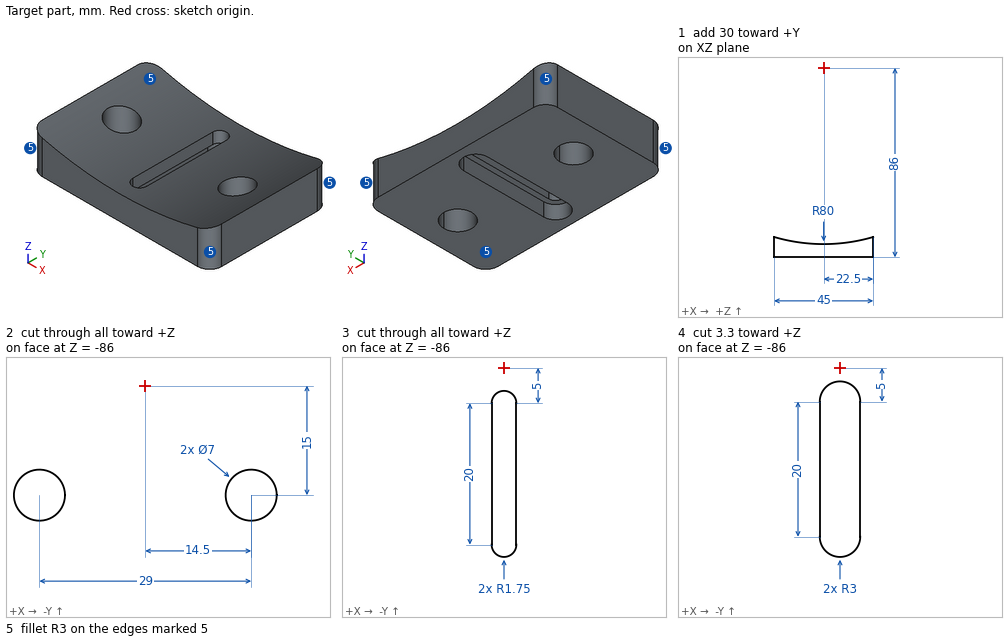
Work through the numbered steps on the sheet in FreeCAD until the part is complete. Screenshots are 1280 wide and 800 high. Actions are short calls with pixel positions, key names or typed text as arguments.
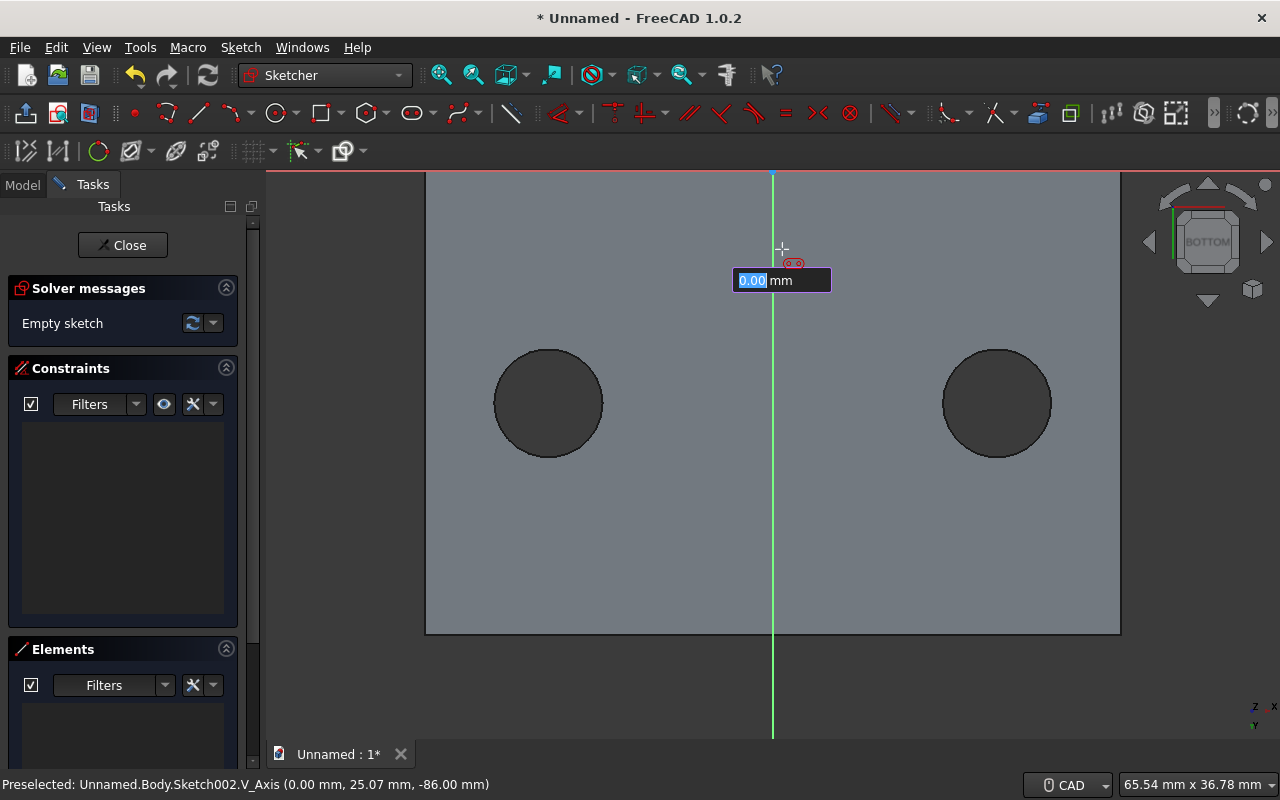
click(746, 403)
key(Escape)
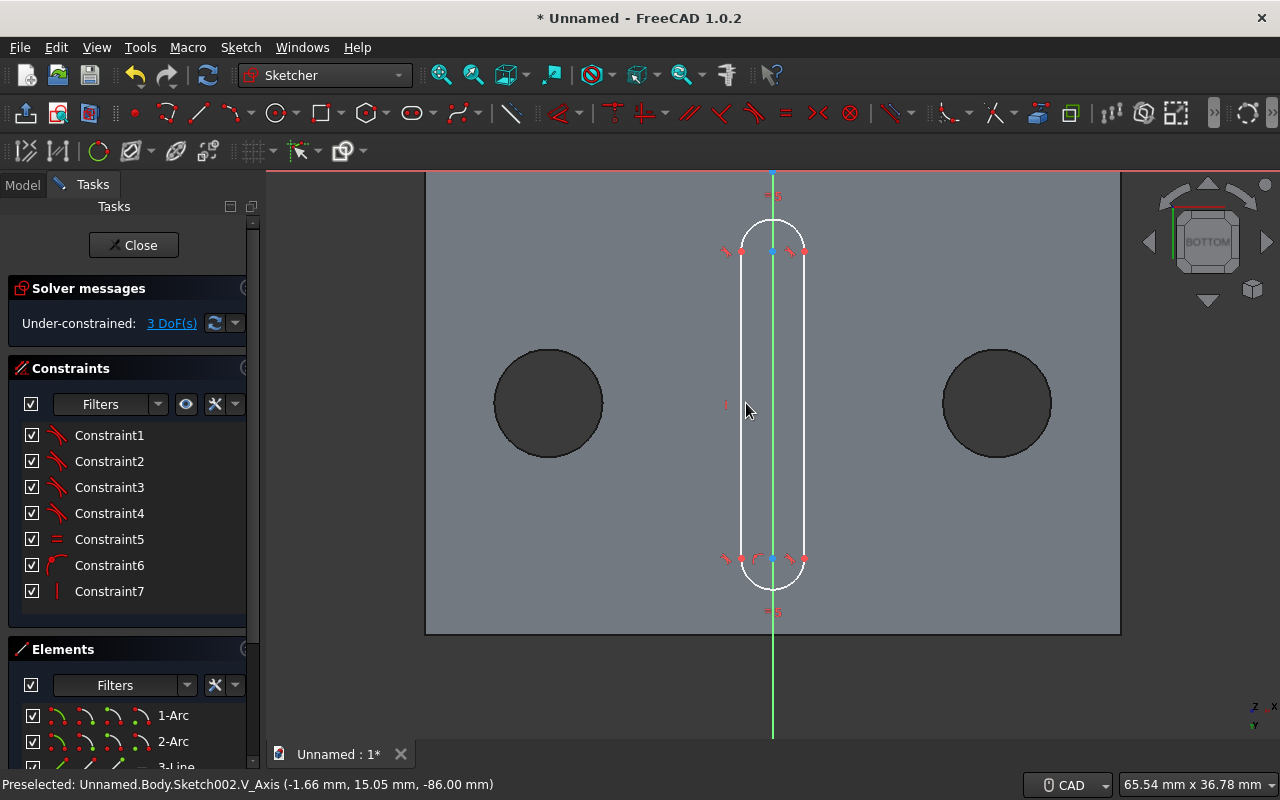
click(558, 114)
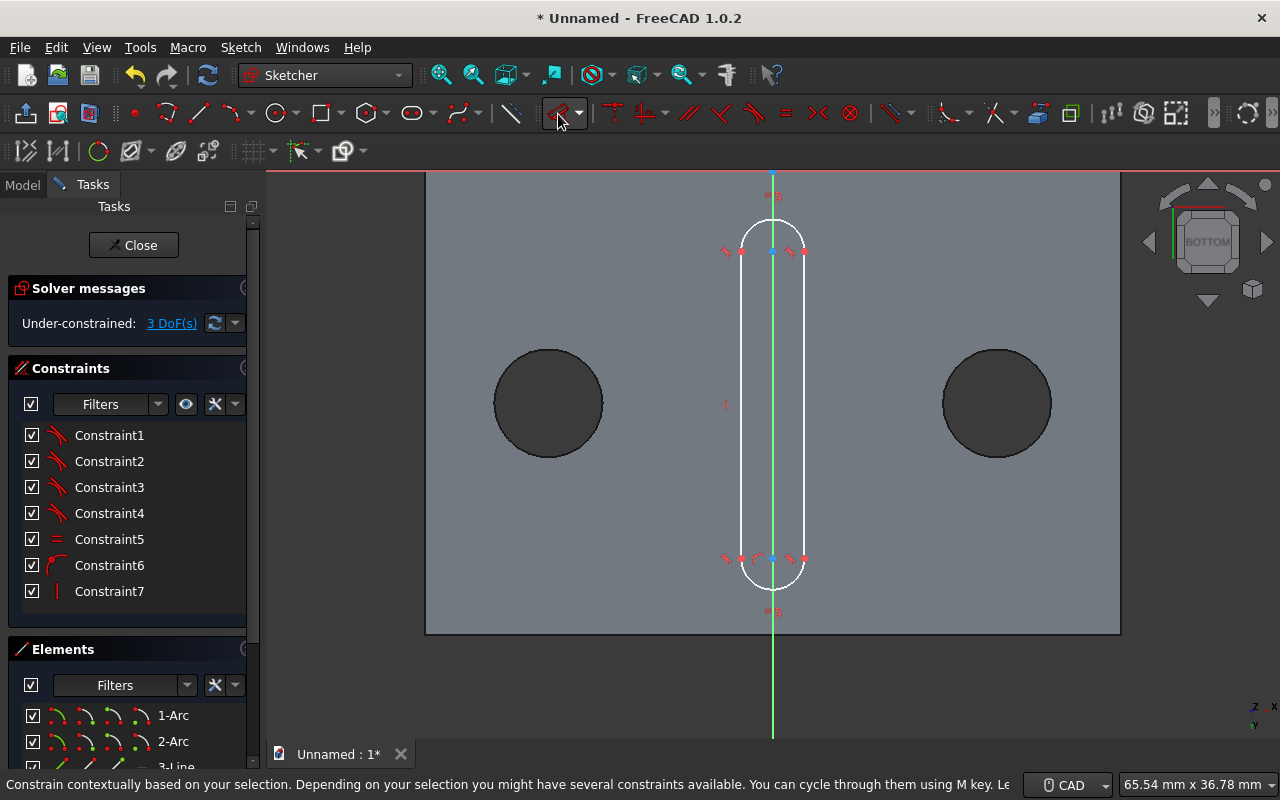
scroll(754, 584, up, 2)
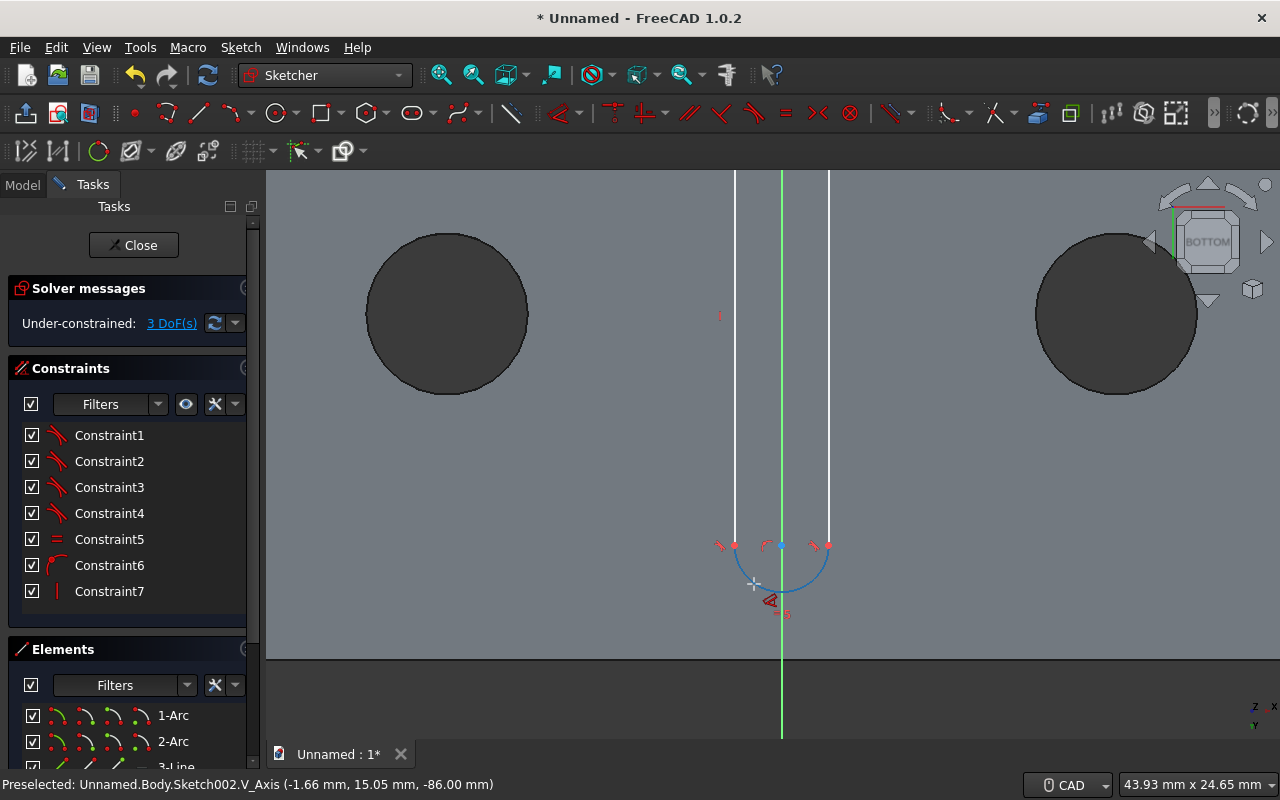
click(754, 583)
click(735, 609)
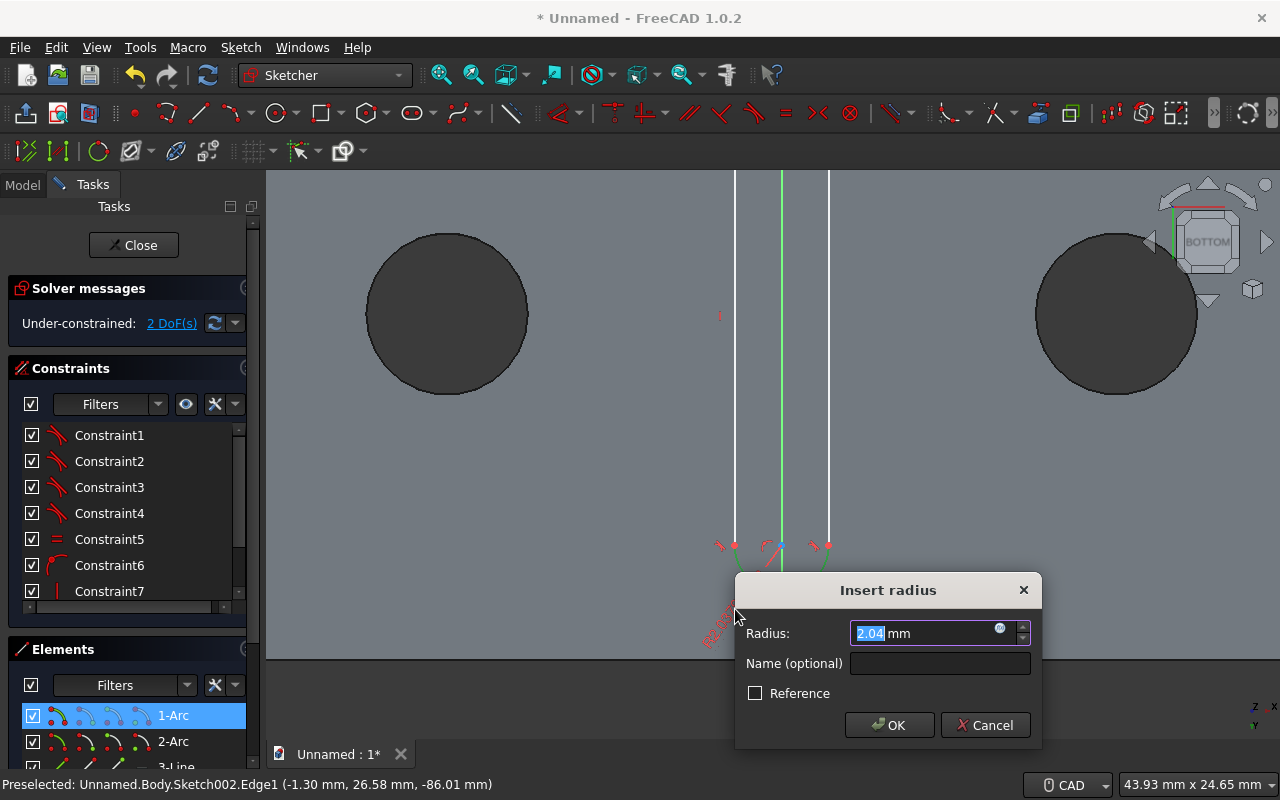
text(1.75)
key(Return)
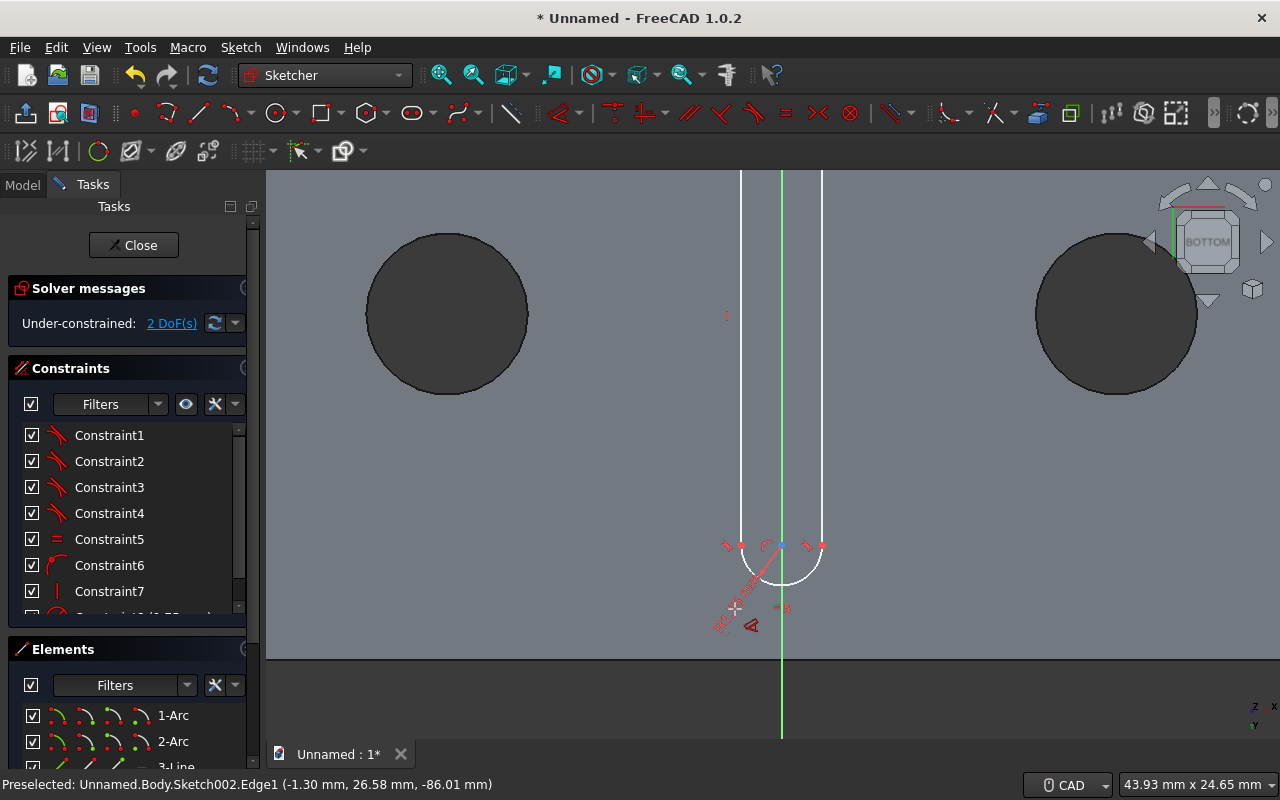
click(741, 408)
click(707, 372)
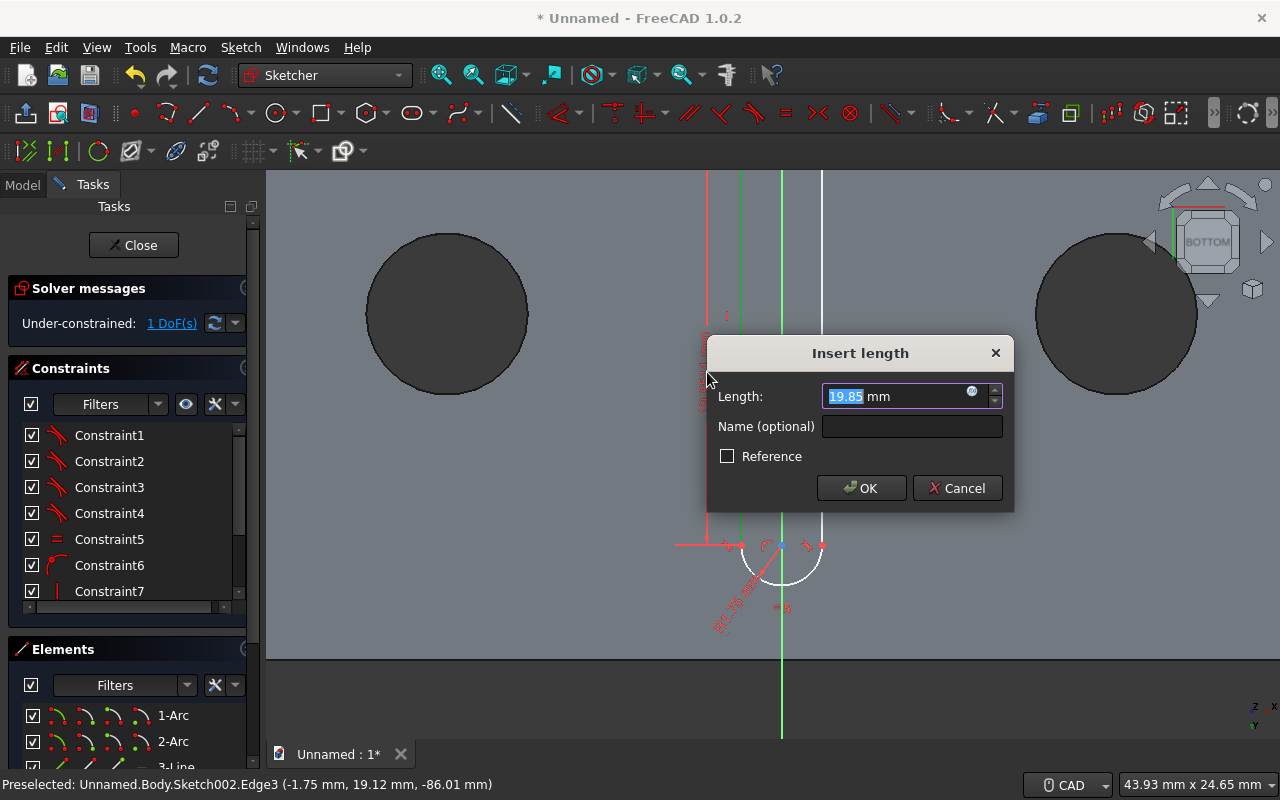
text(20)
key(Return)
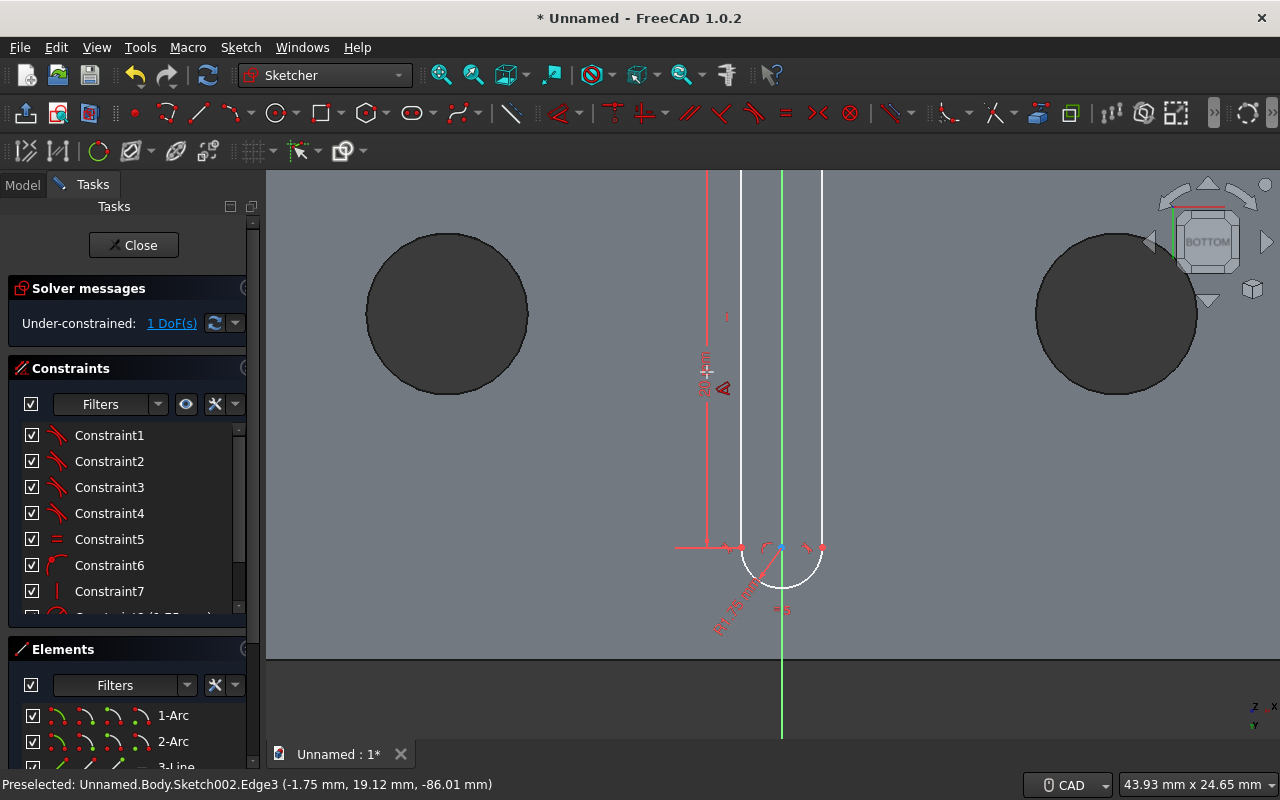
scroll(611, 671, down, 3)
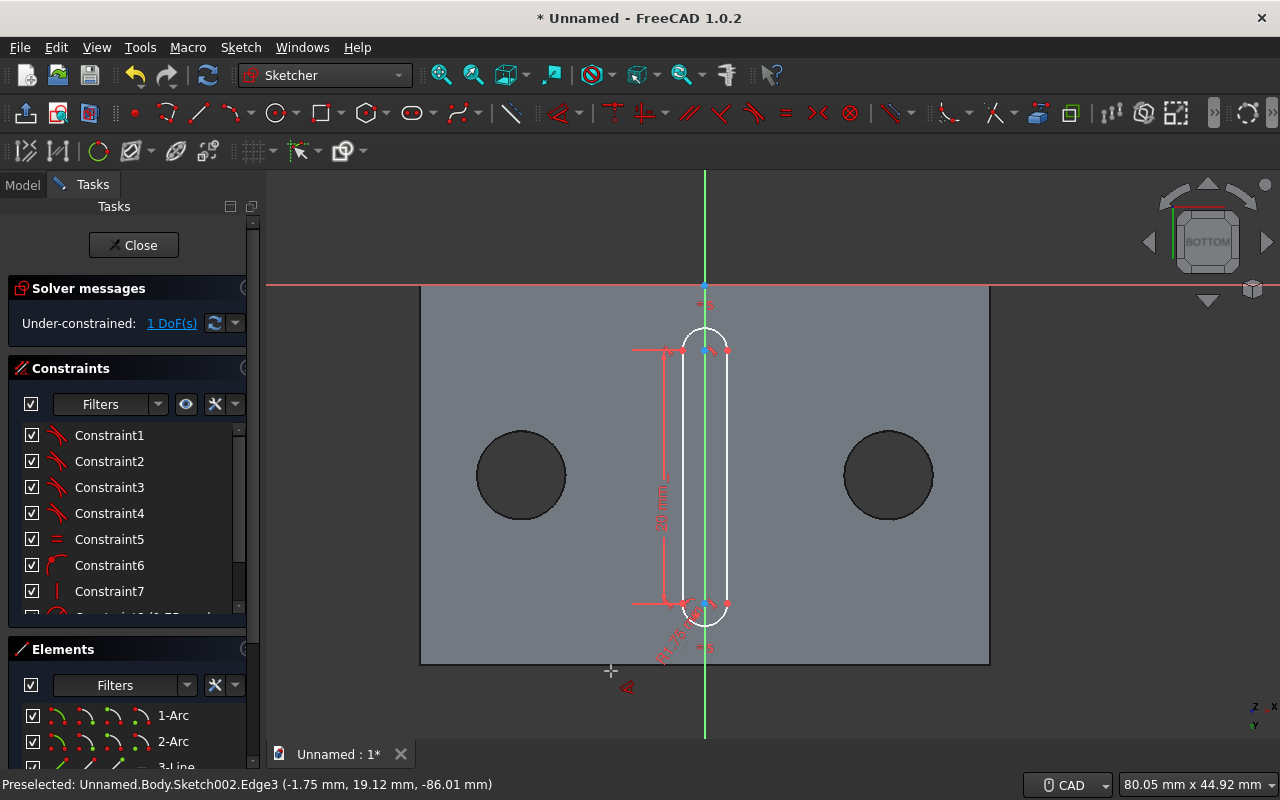
click(727, 350)
click(761, 318)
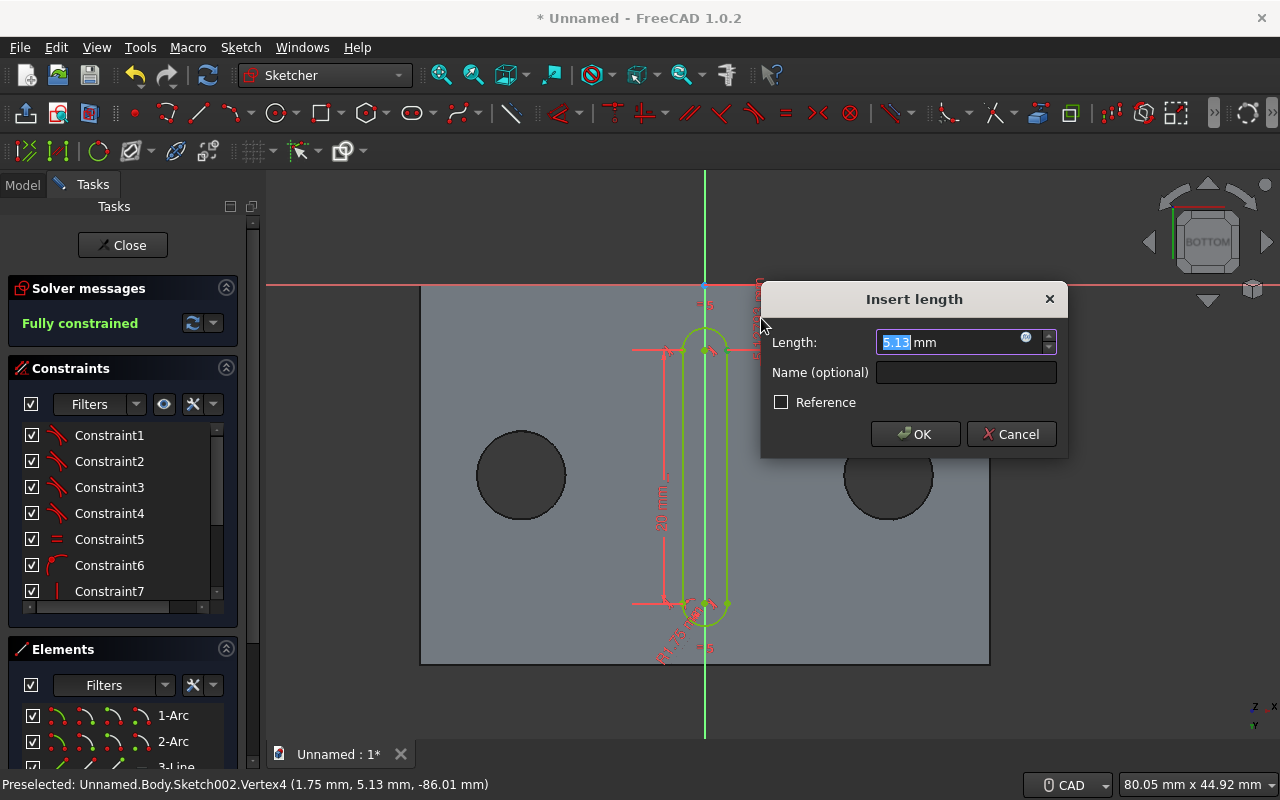
text(5)
key(Return)
key(Escape)